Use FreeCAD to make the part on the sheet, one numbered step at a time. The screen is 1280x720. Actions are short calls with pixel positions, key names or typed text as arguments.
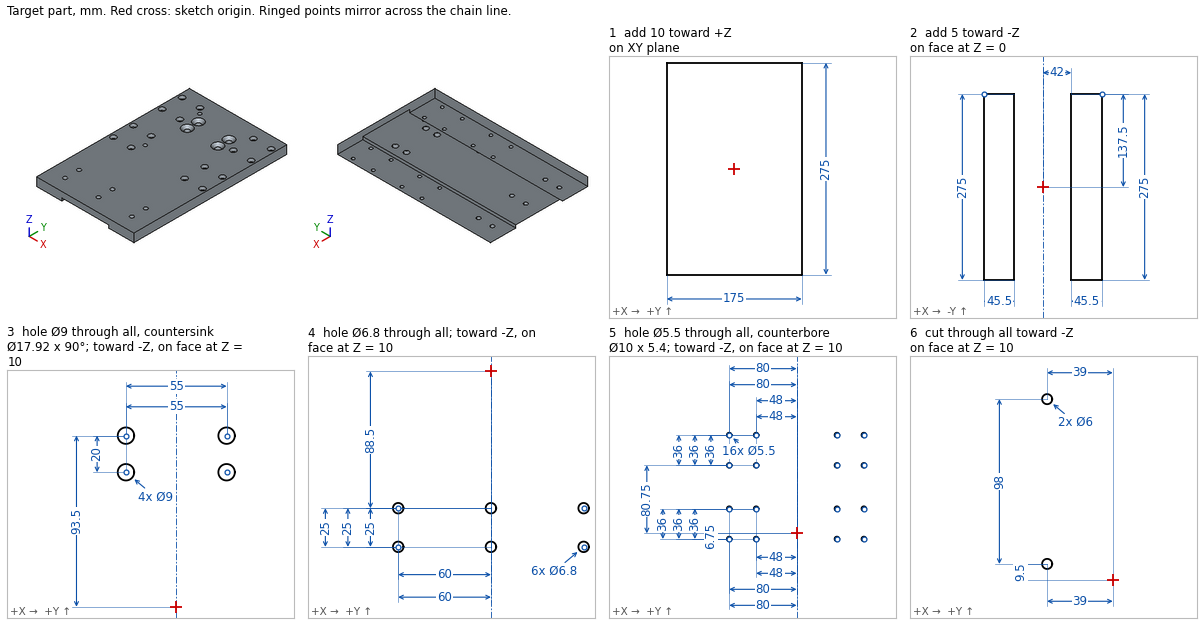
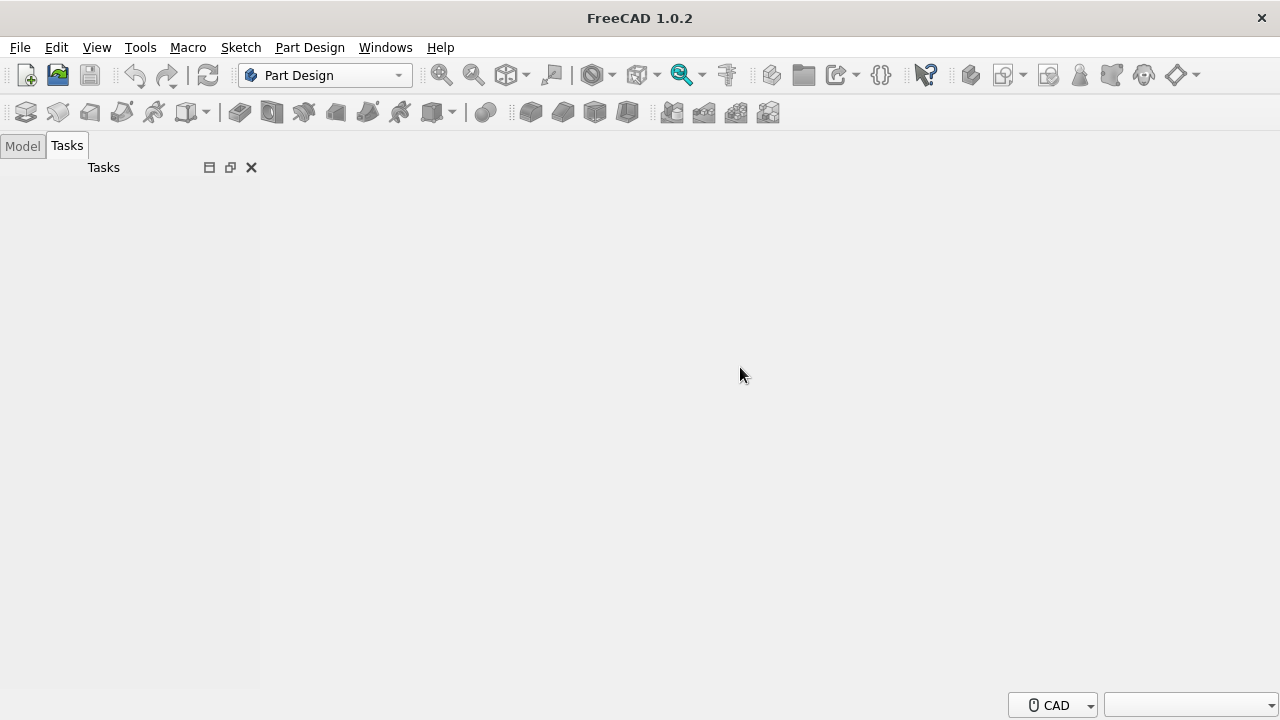
key(ctrl+n)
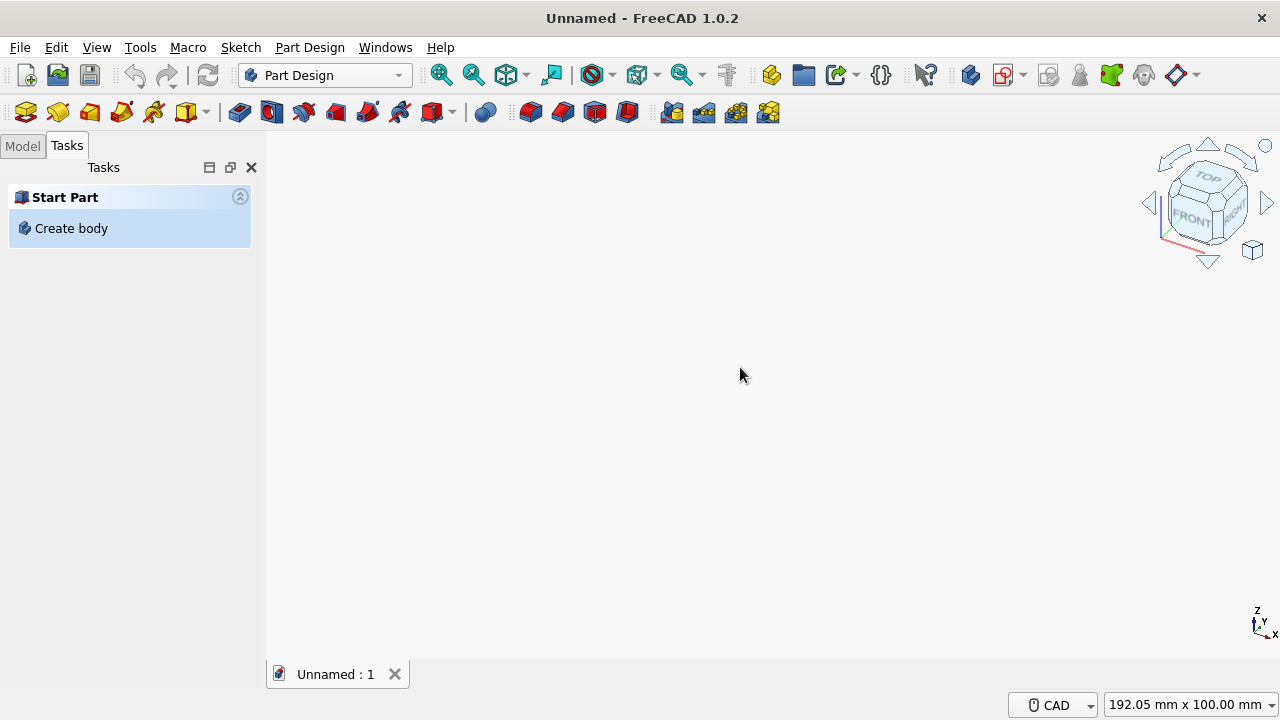
click(1004, 76)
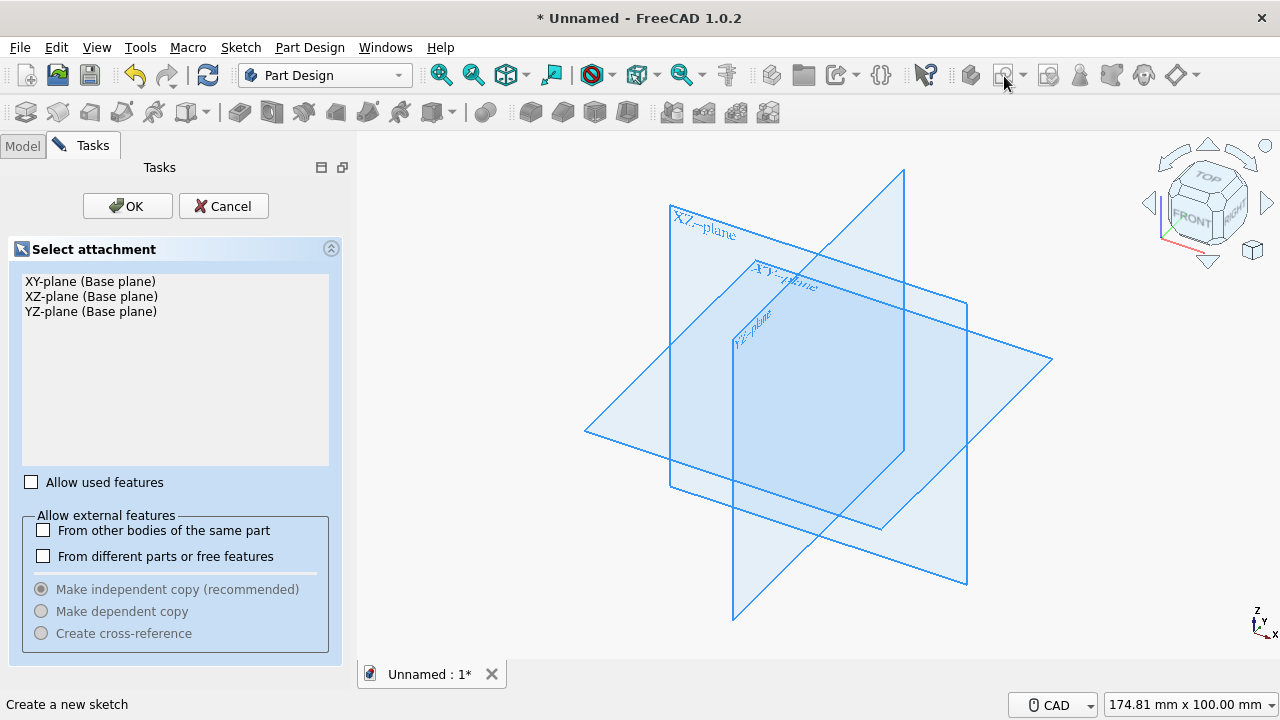
click(82, 282)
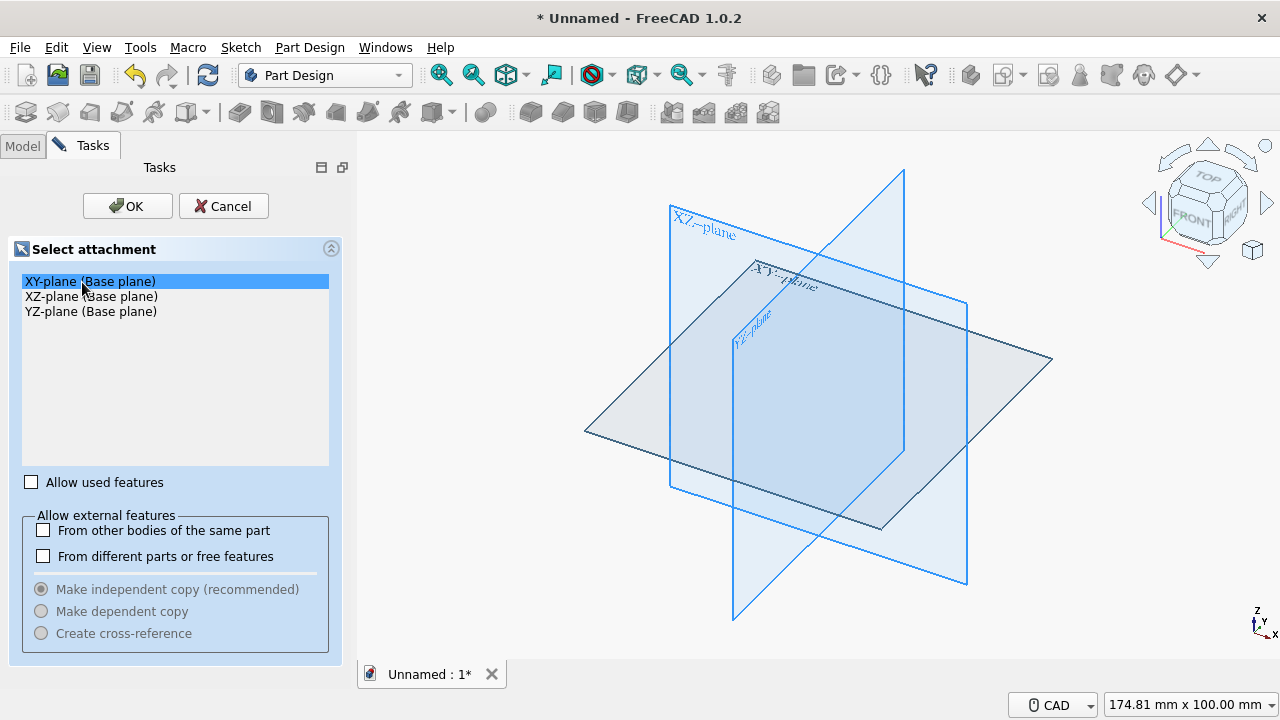
click(128, 206)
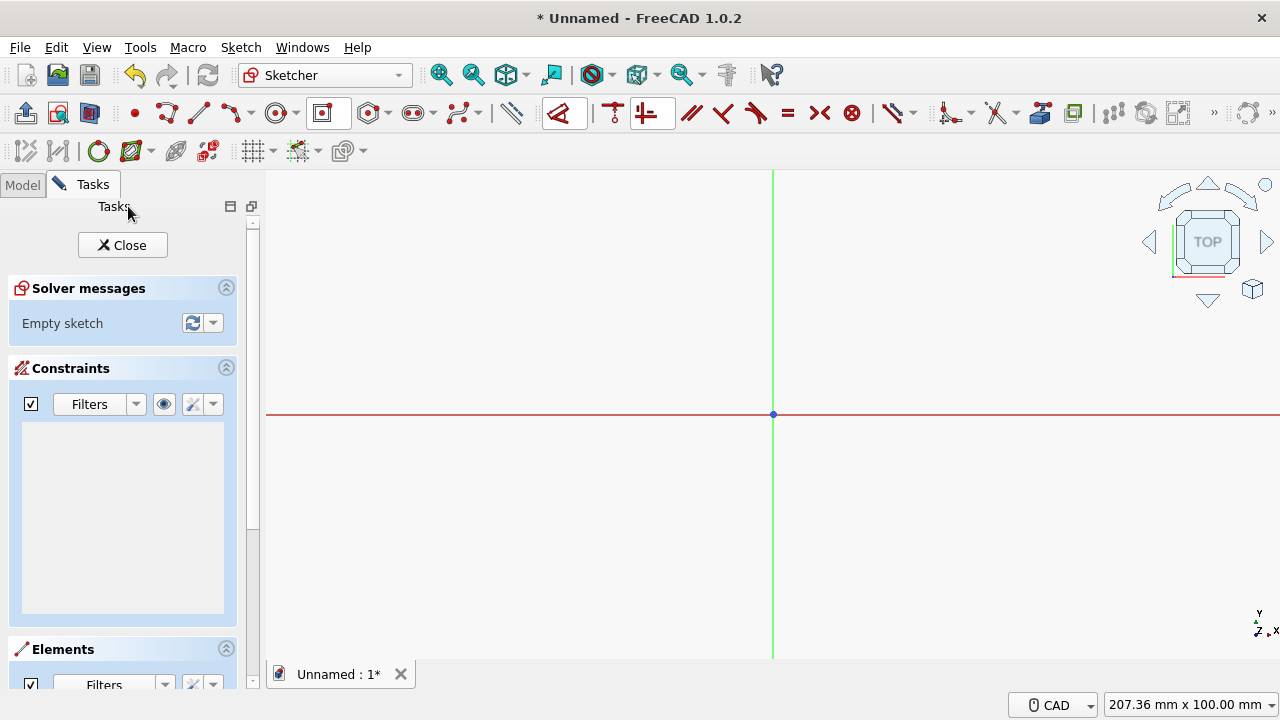
scroll(682, 415, down, 7)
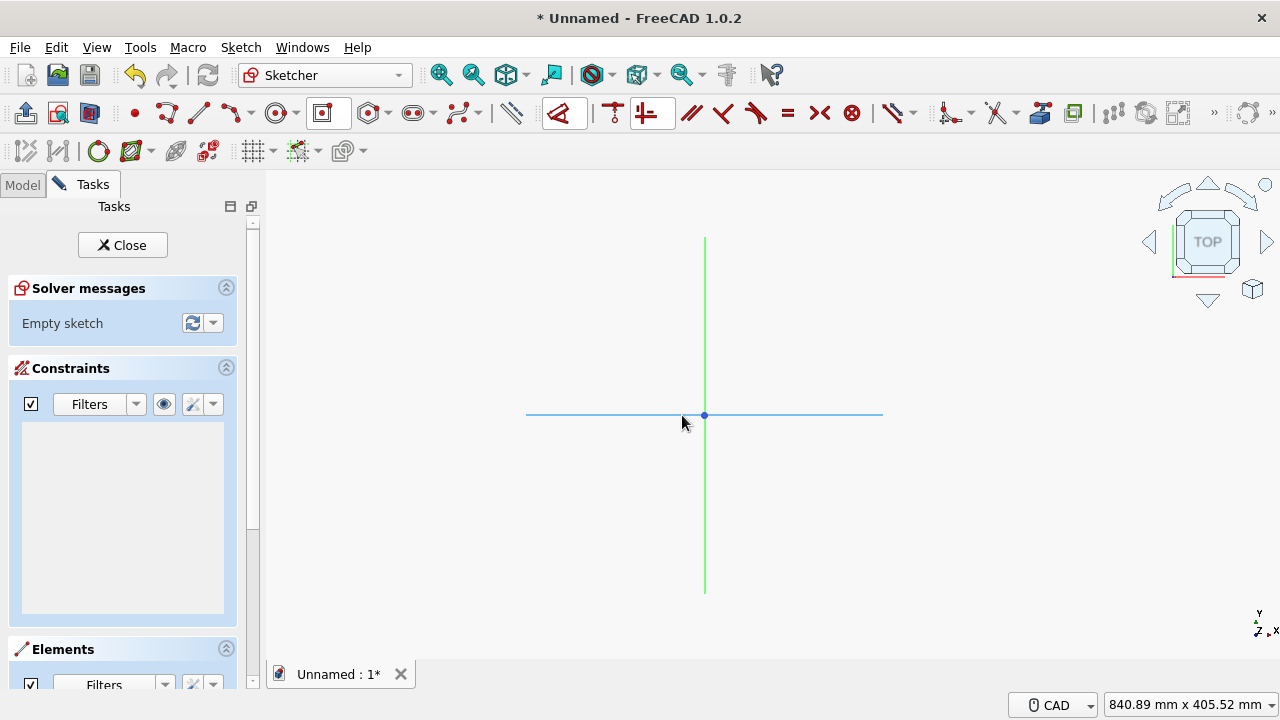
click(322, 114)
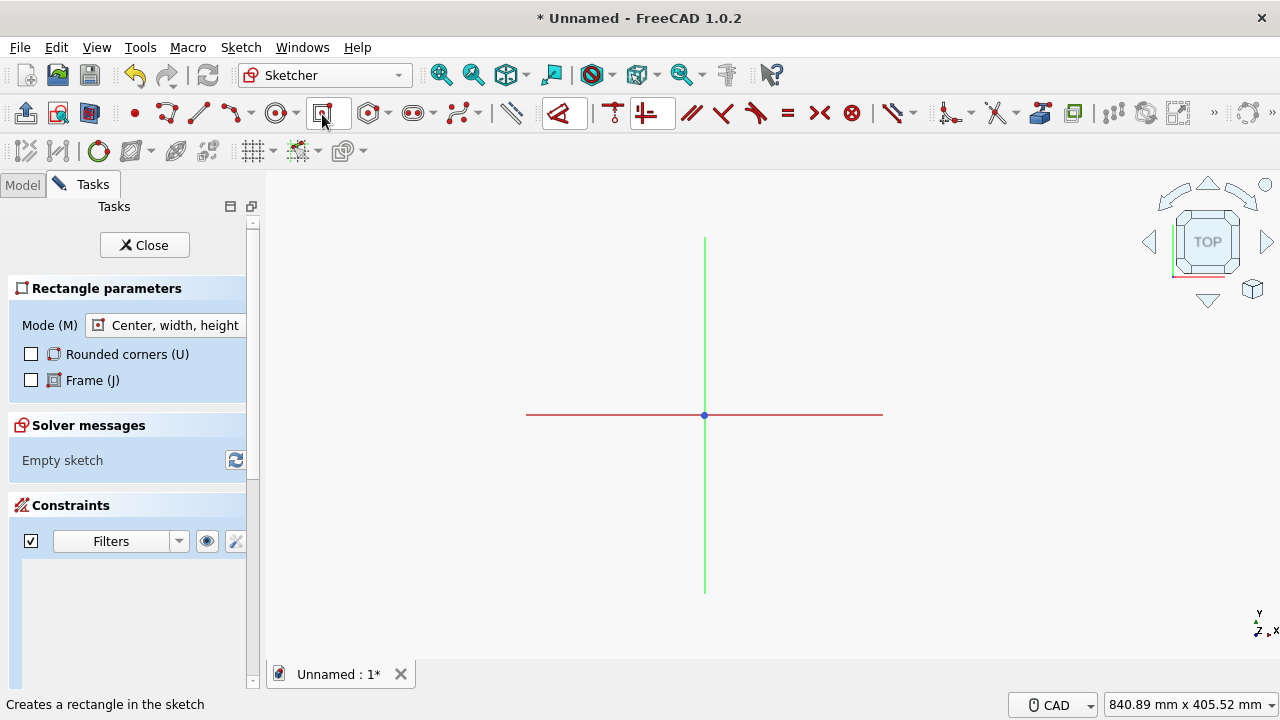
click(705, 415)
move(810, 249)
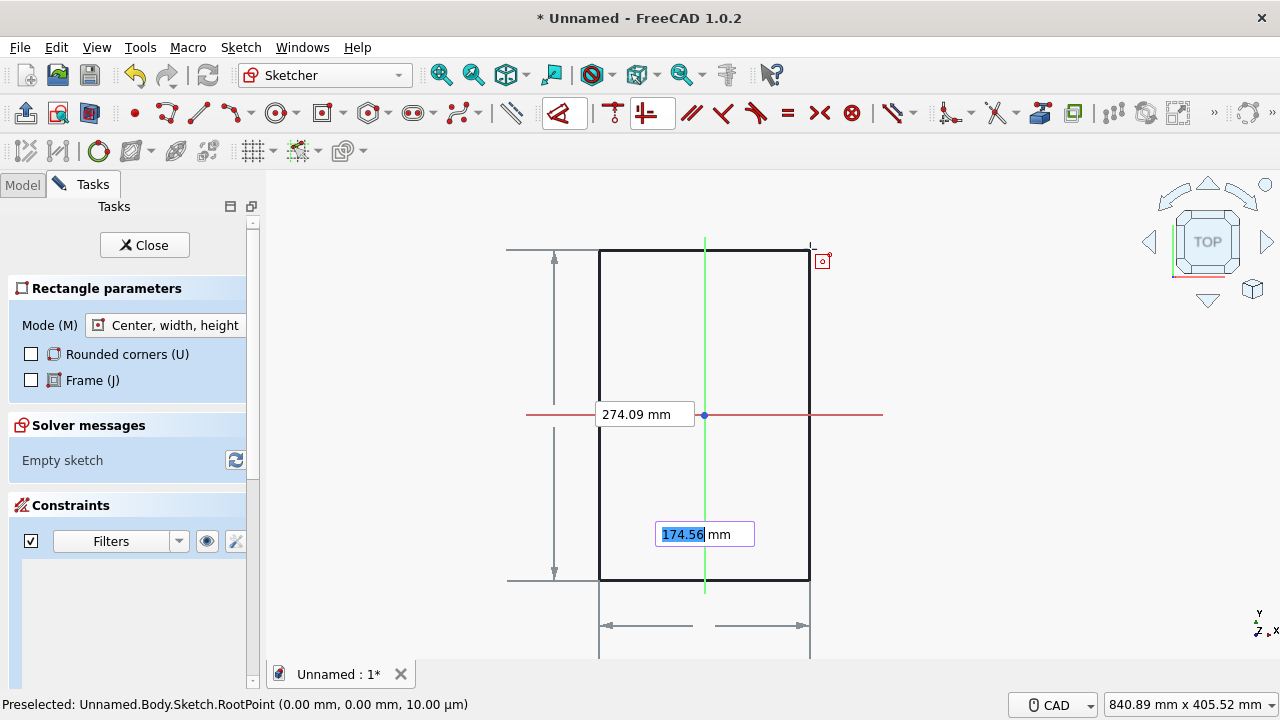
text(175)
key(Tab)
text(275)
key(Return)
key(Escape)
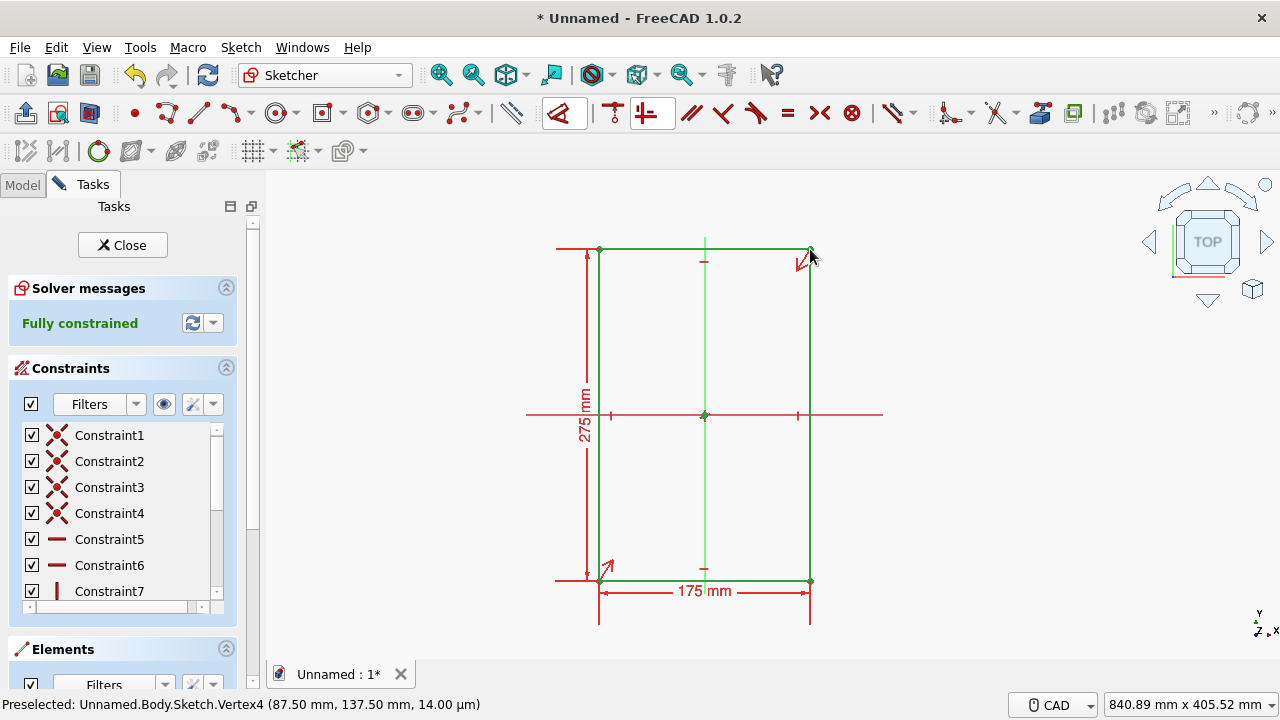
click(123, 245)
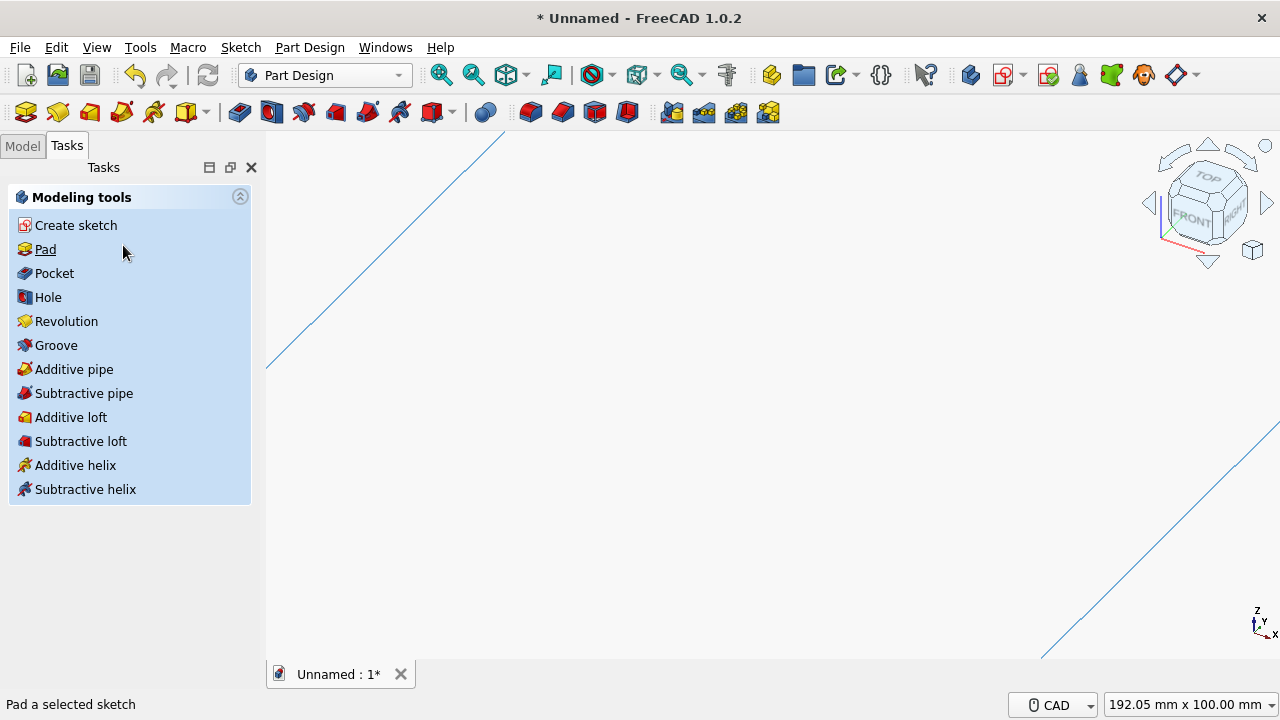
click(26, 112)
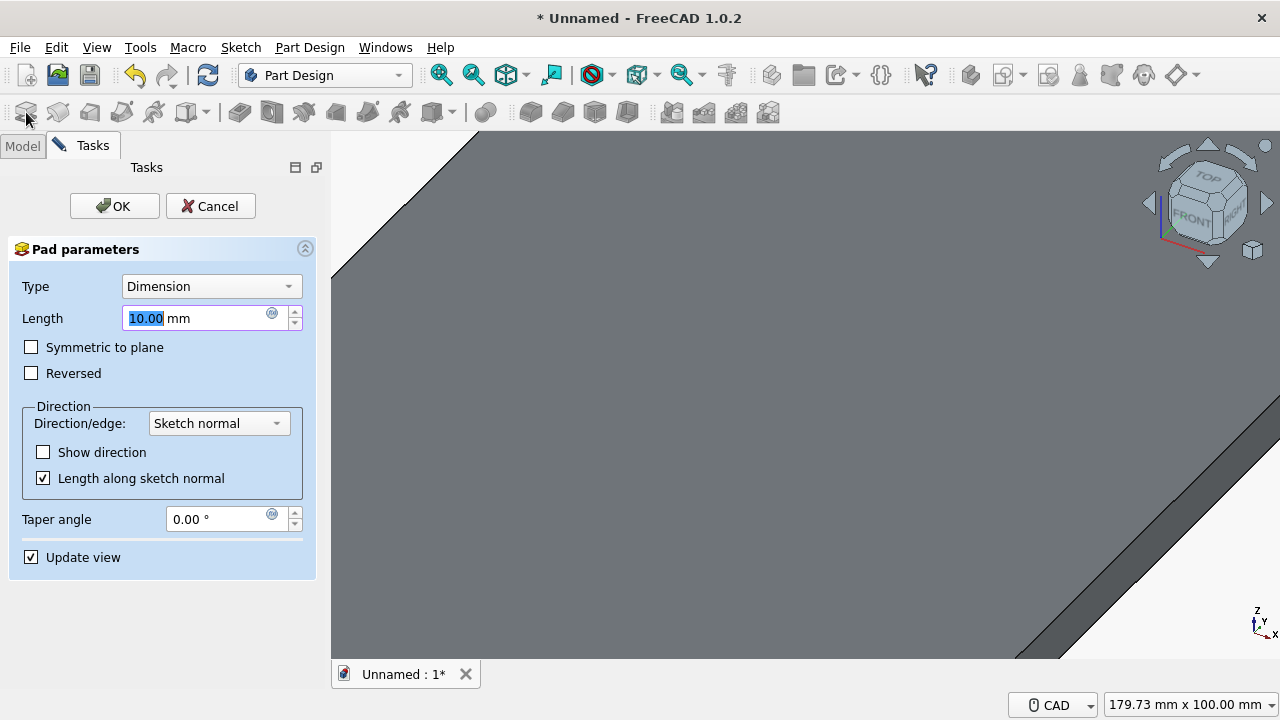
text(10)
key(Tab)